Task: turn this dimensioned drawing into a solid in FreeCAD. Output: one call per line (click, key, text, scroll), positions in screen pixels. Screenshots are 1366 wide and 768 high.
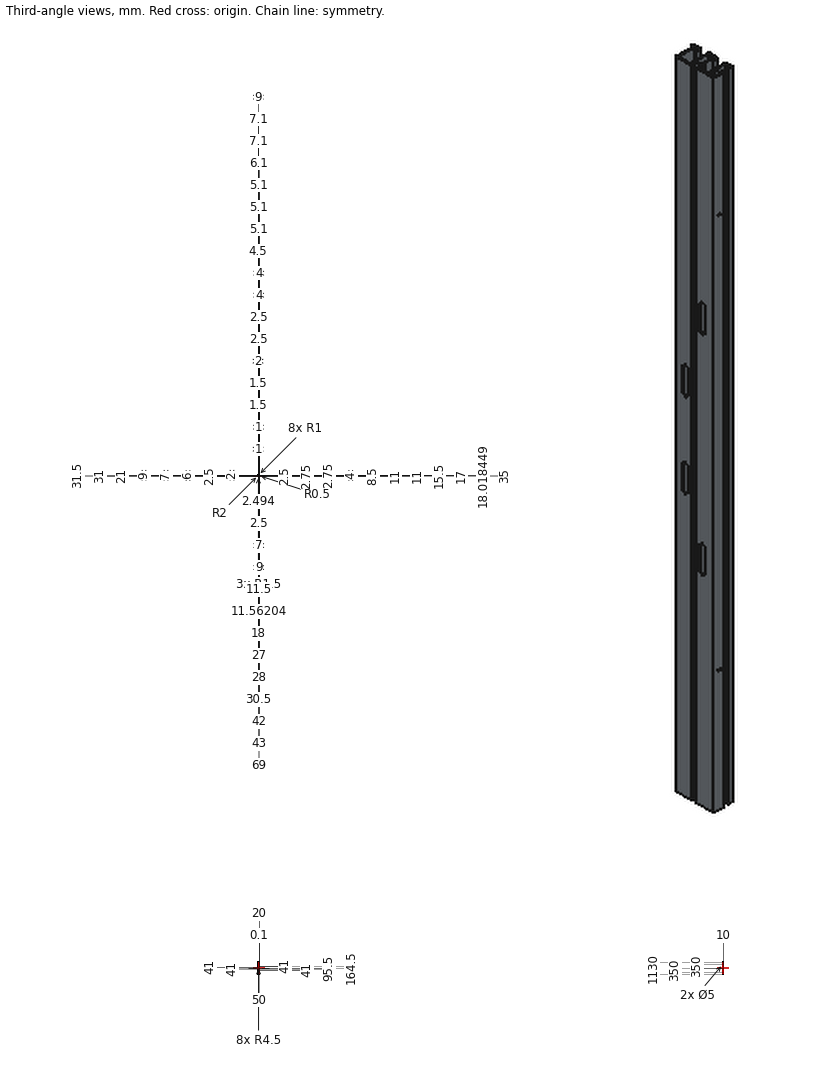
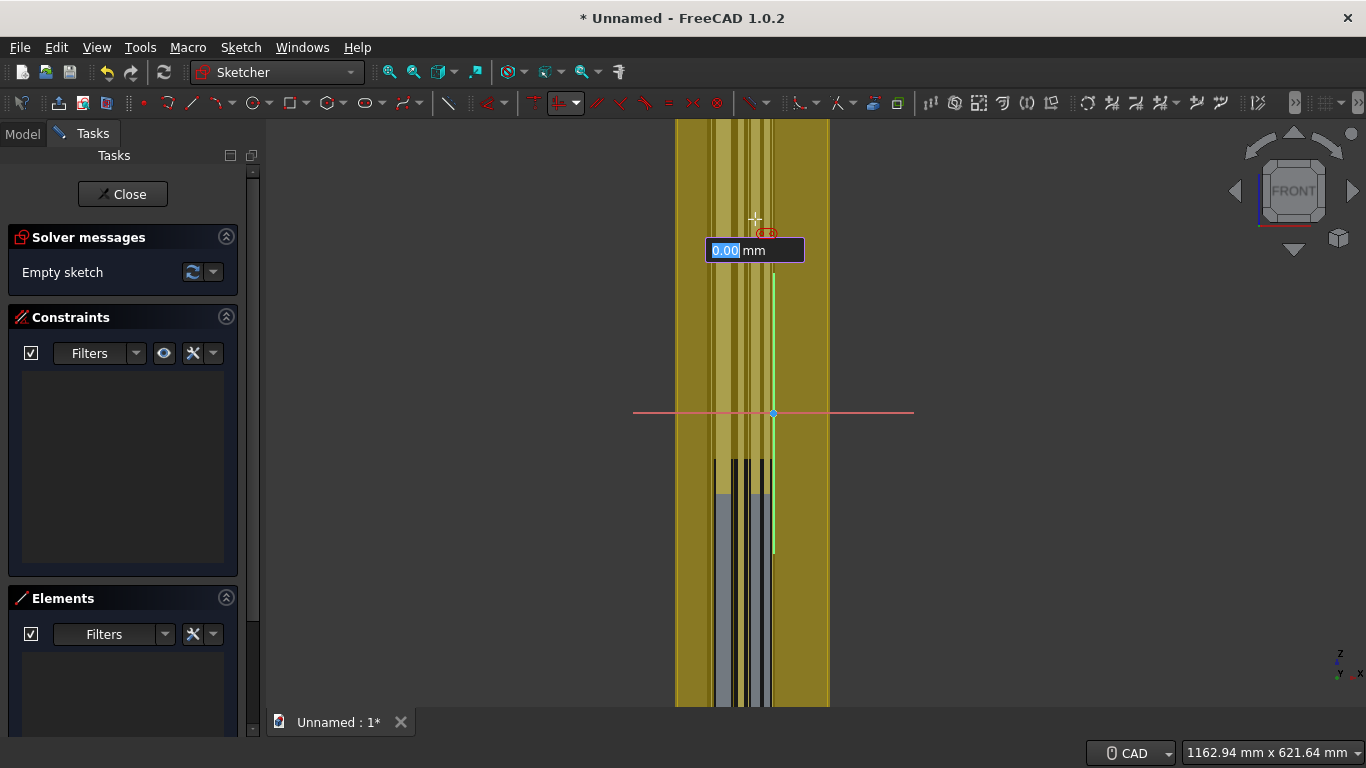
scroll(759, 238, up, 7)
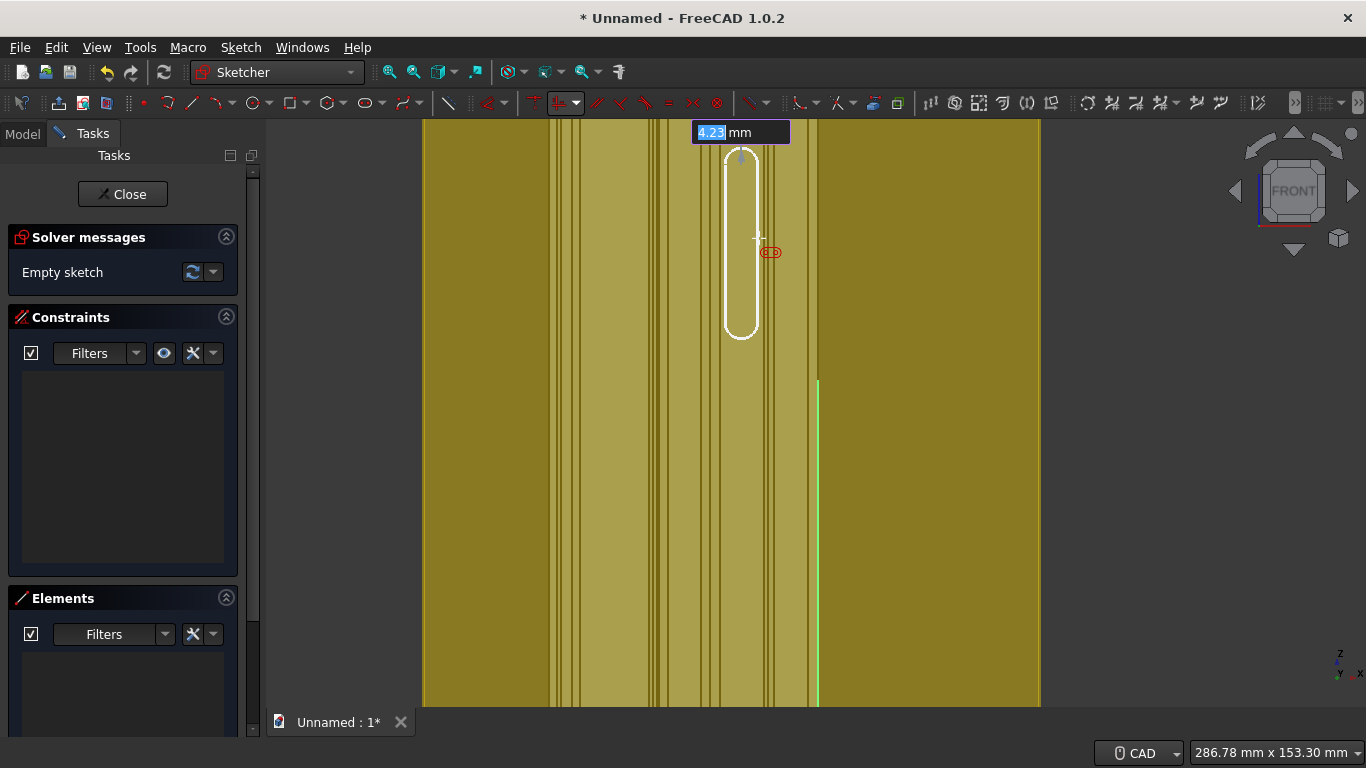
click(758, 239)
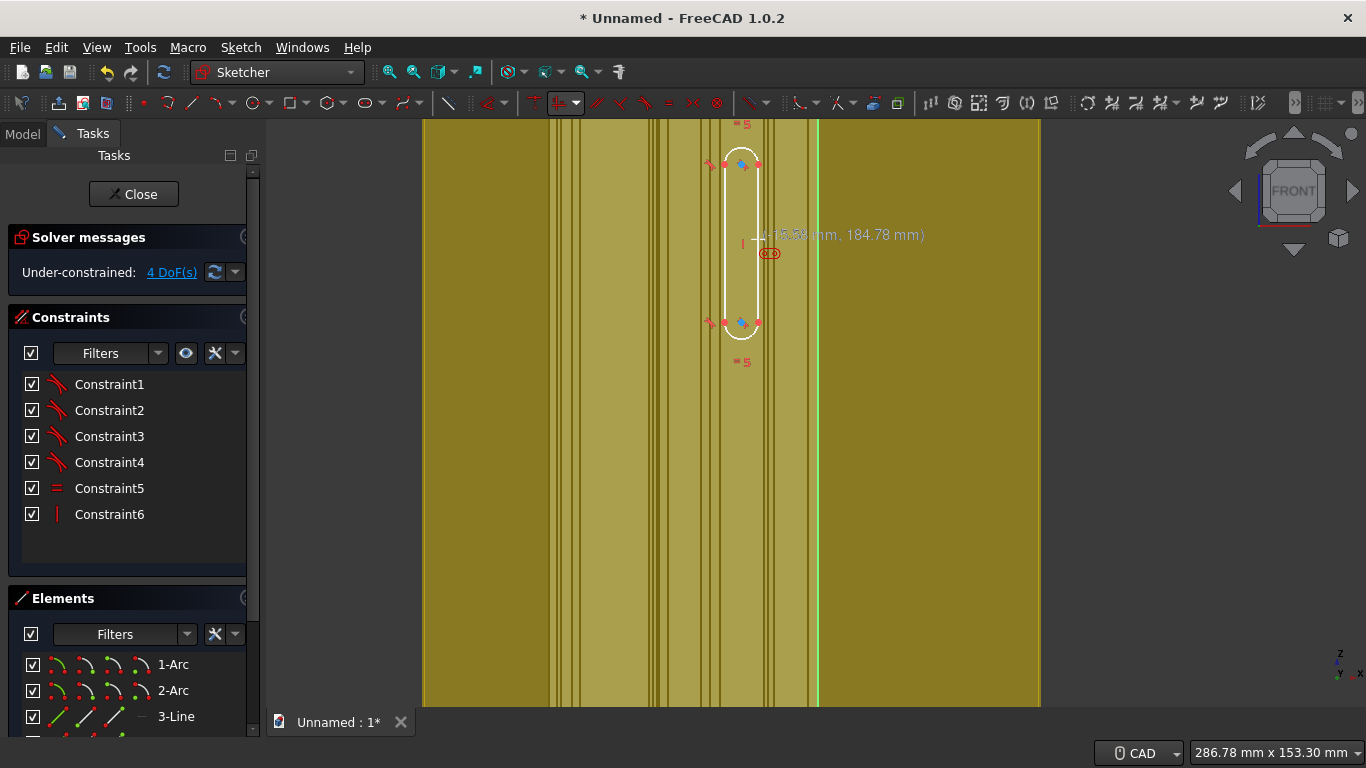
scroll(759, 238, down, 7)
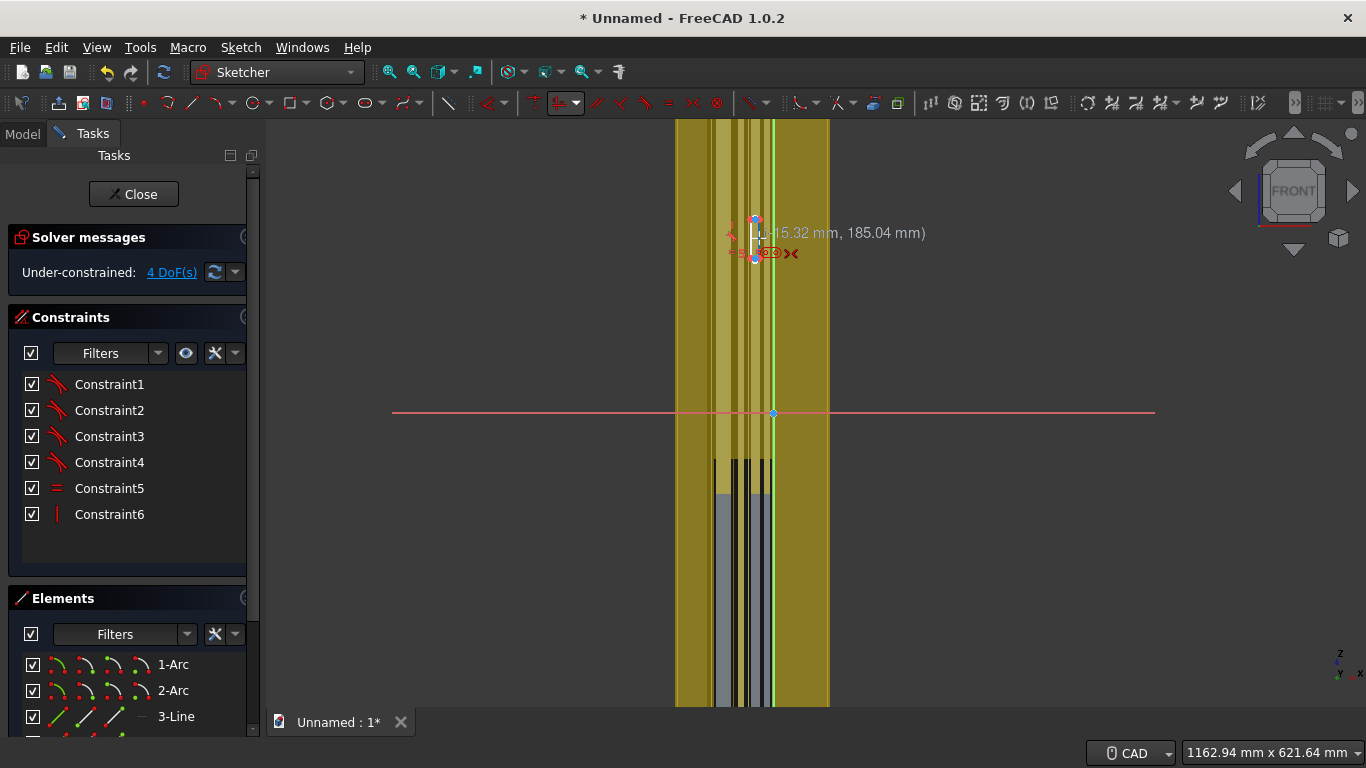
scroll(727, 504, up, 9)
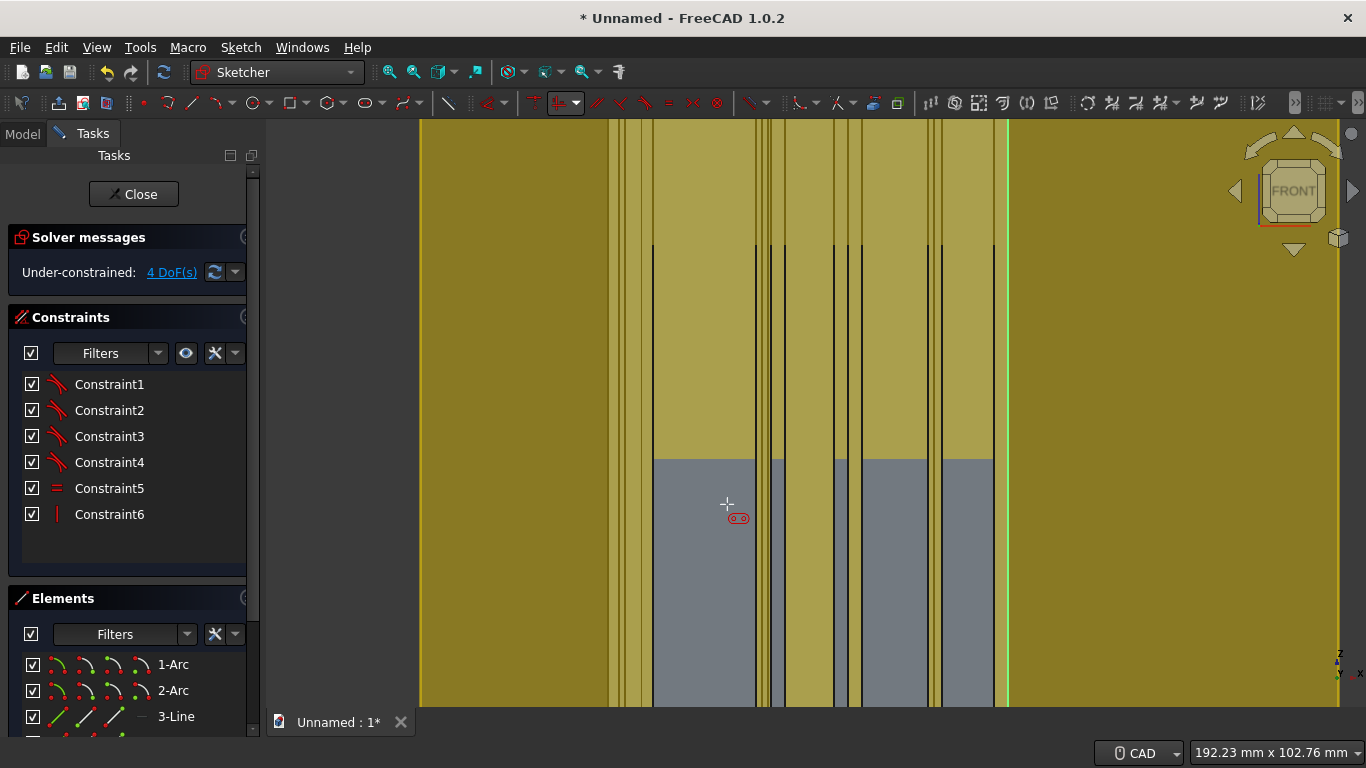
scroll(727, 504, down, 9)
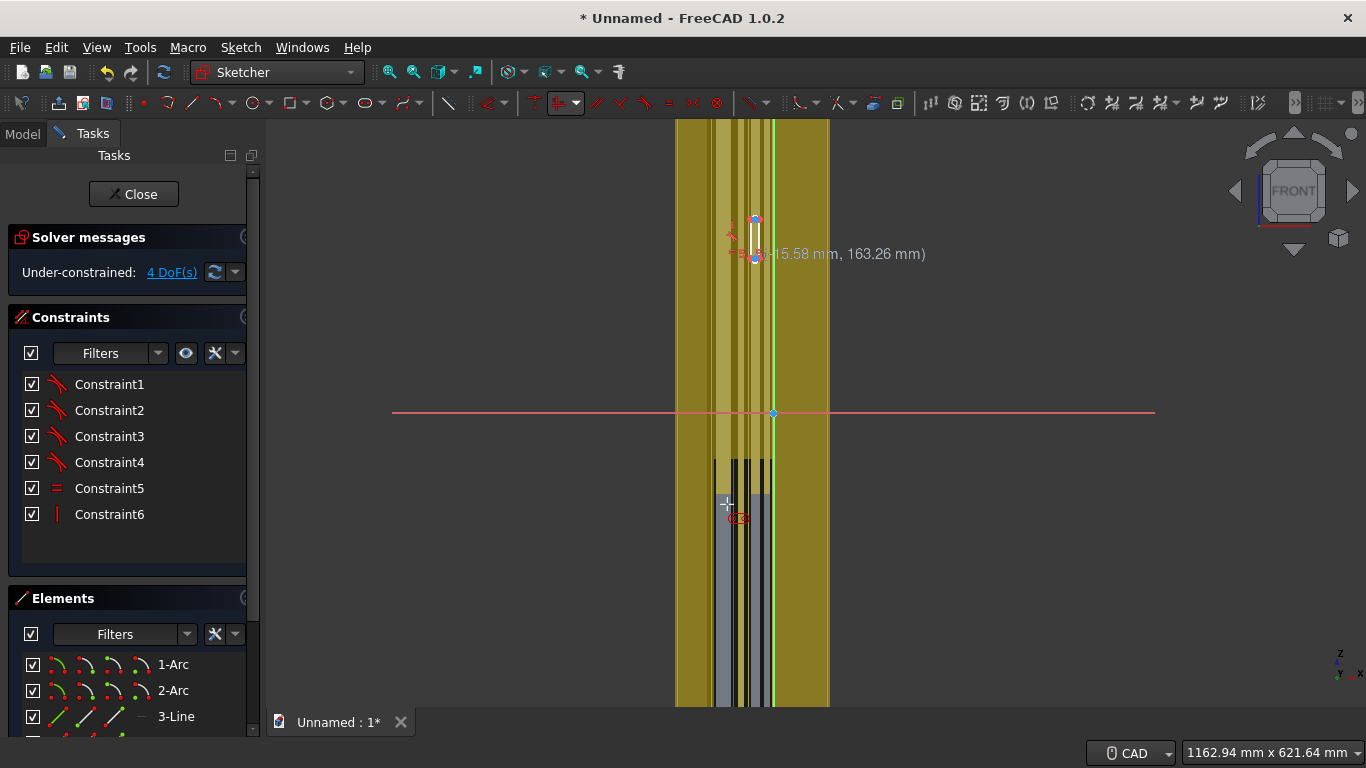
click(727, 504)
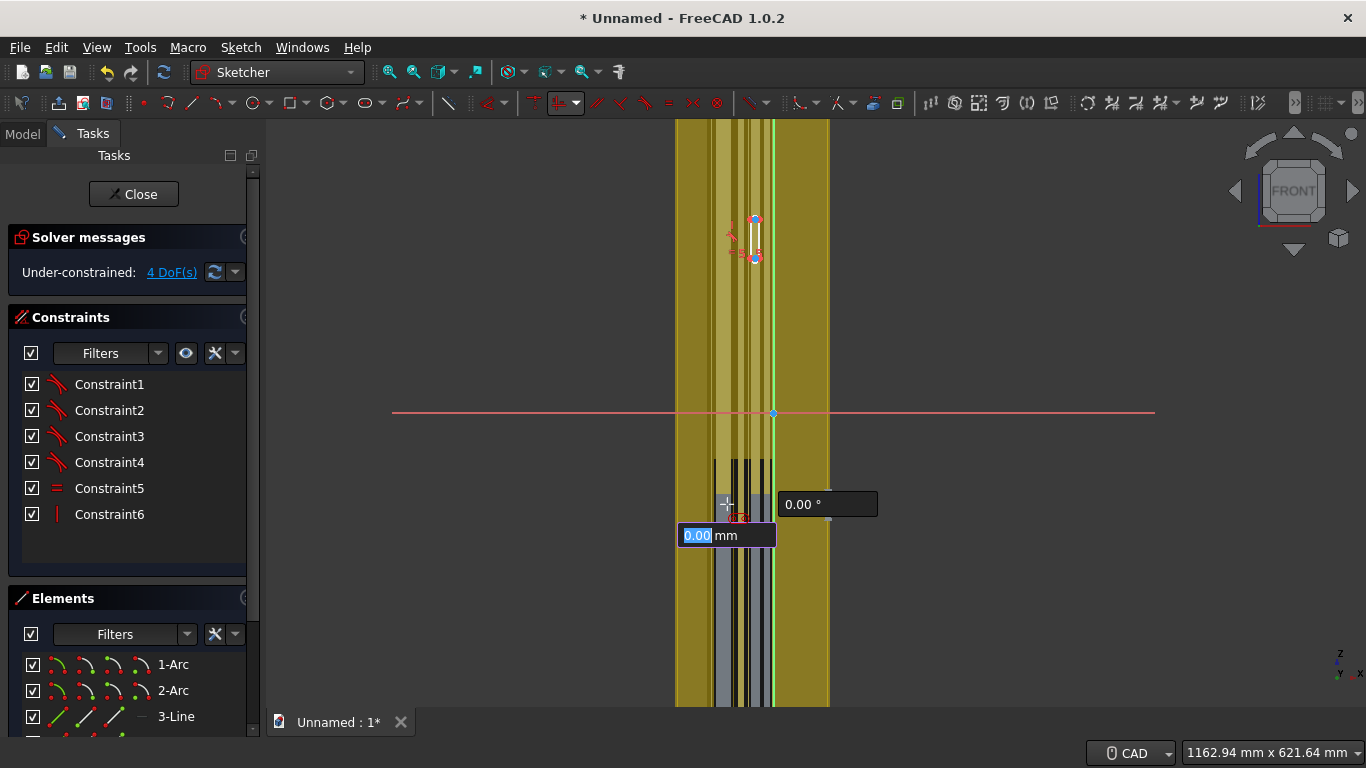
click(727, 465)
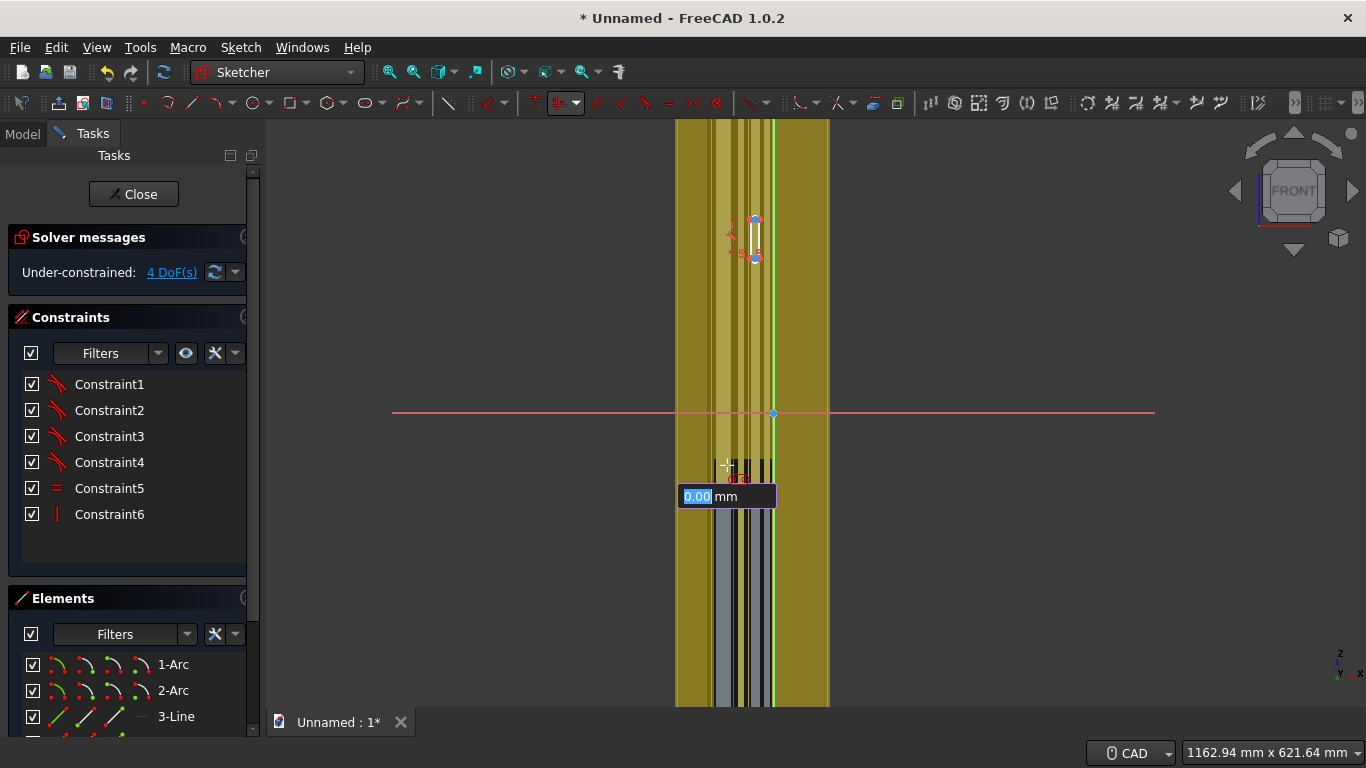
scroll(731, 484, up, 7)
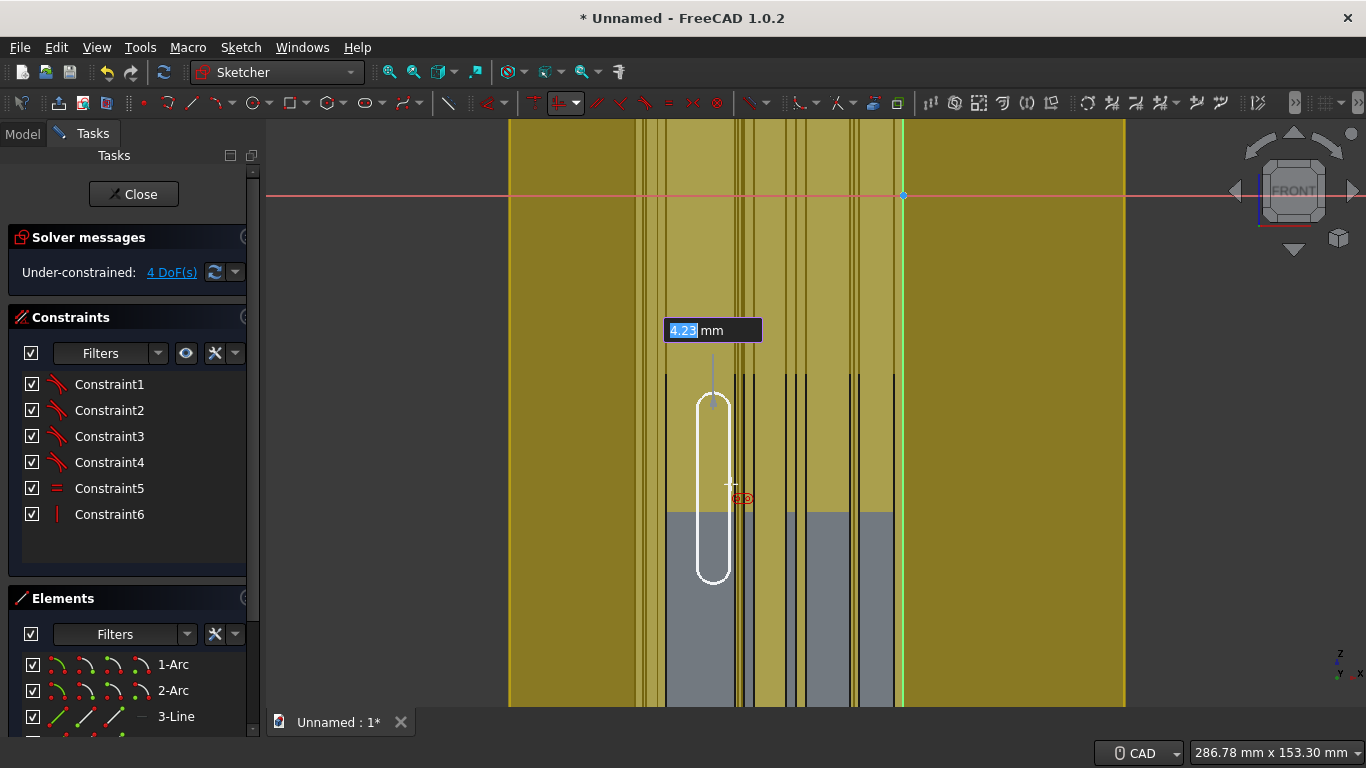
click(729, 484)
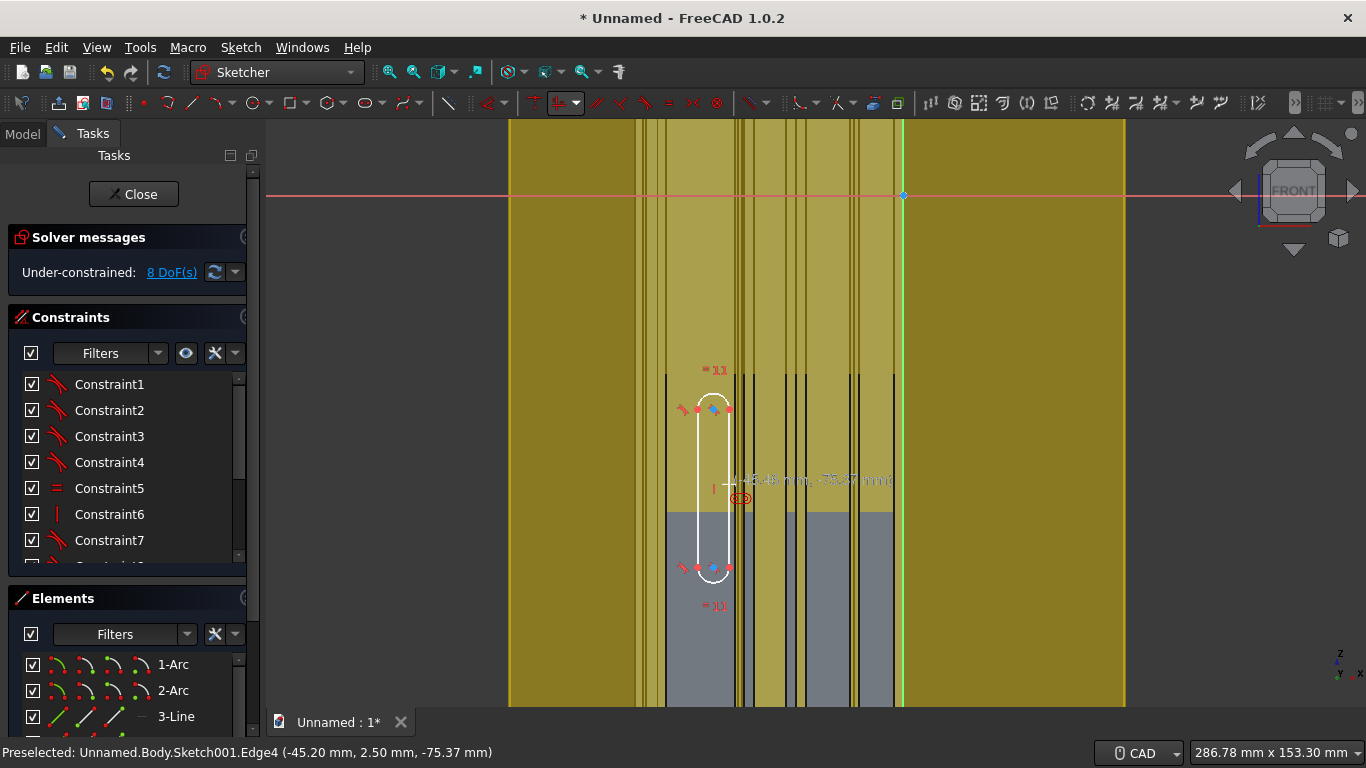
scroll(731, 484, down, 7)